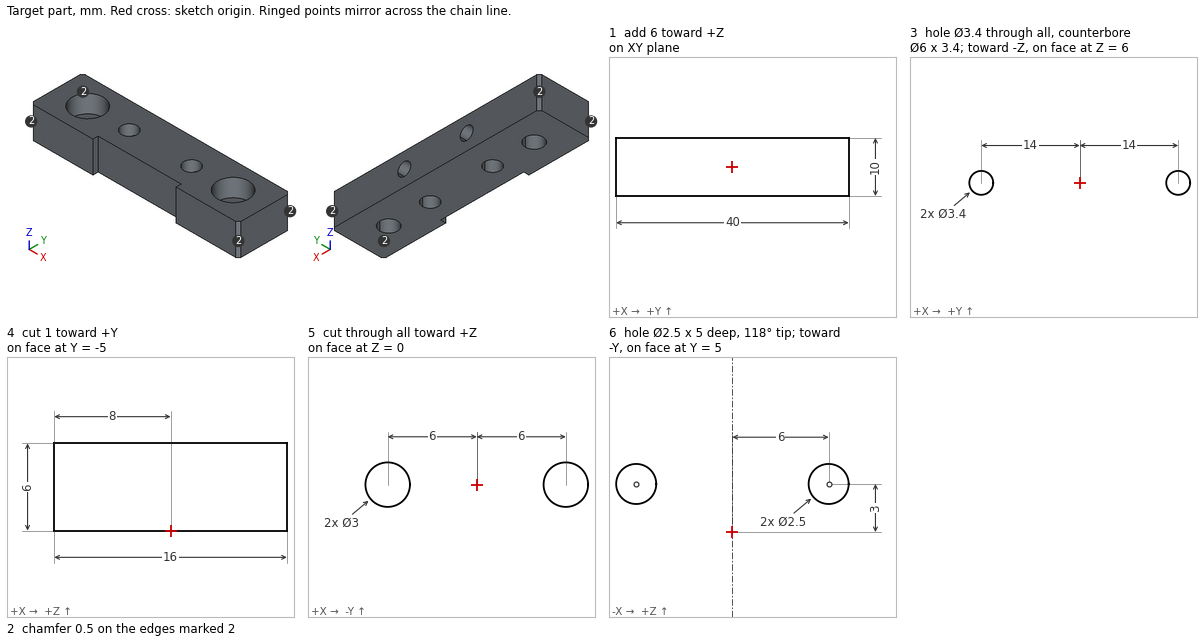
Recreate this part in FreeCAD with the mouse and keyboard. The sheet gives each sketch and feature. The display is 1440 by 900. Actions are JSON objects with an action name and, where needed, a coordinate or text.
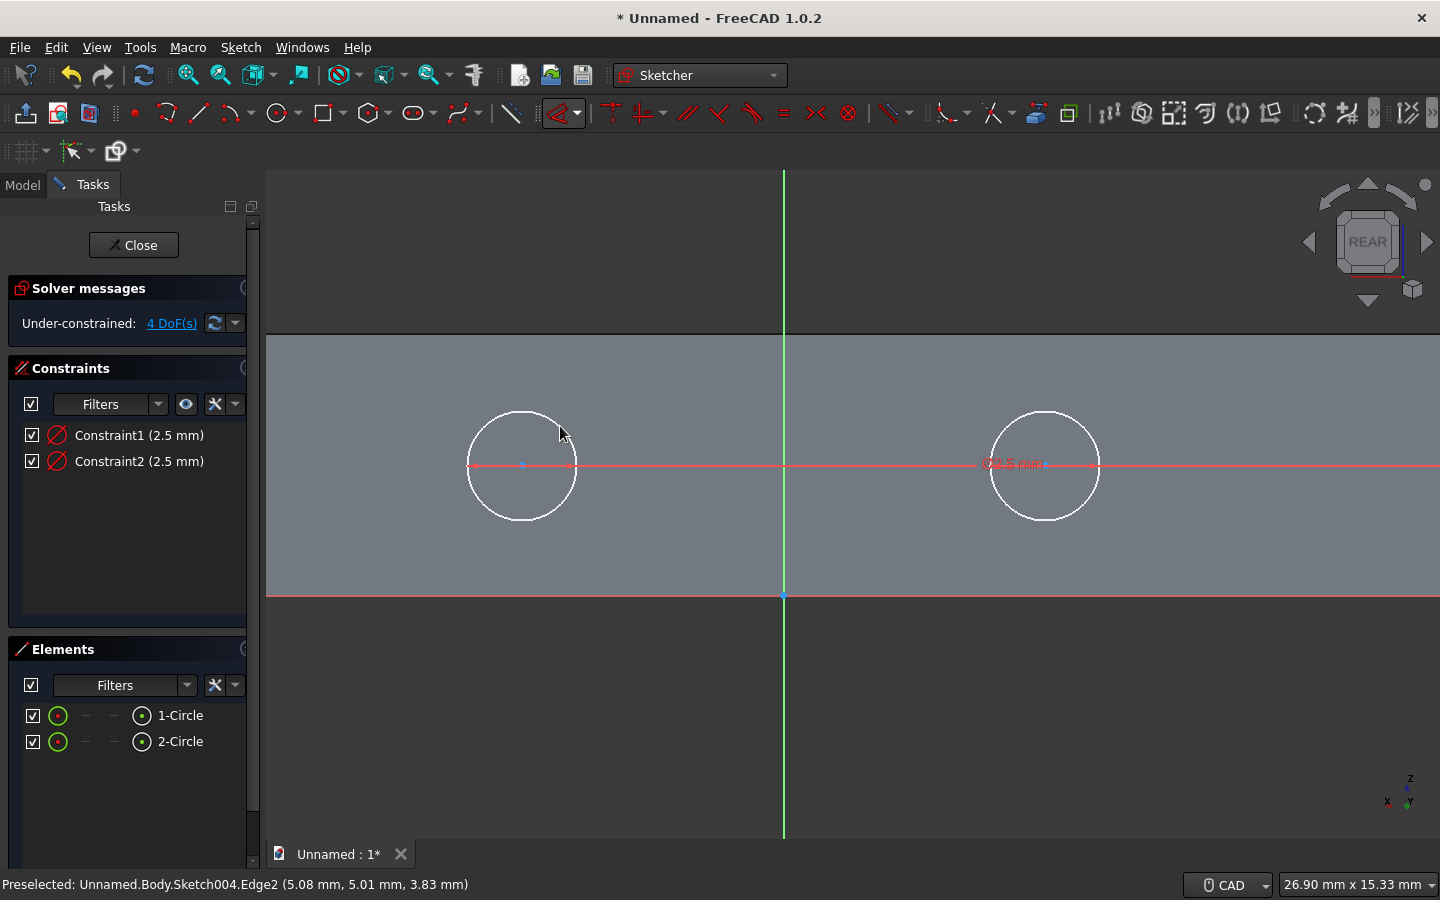
{"action": "left_click", "coordinate": [1045, 466]}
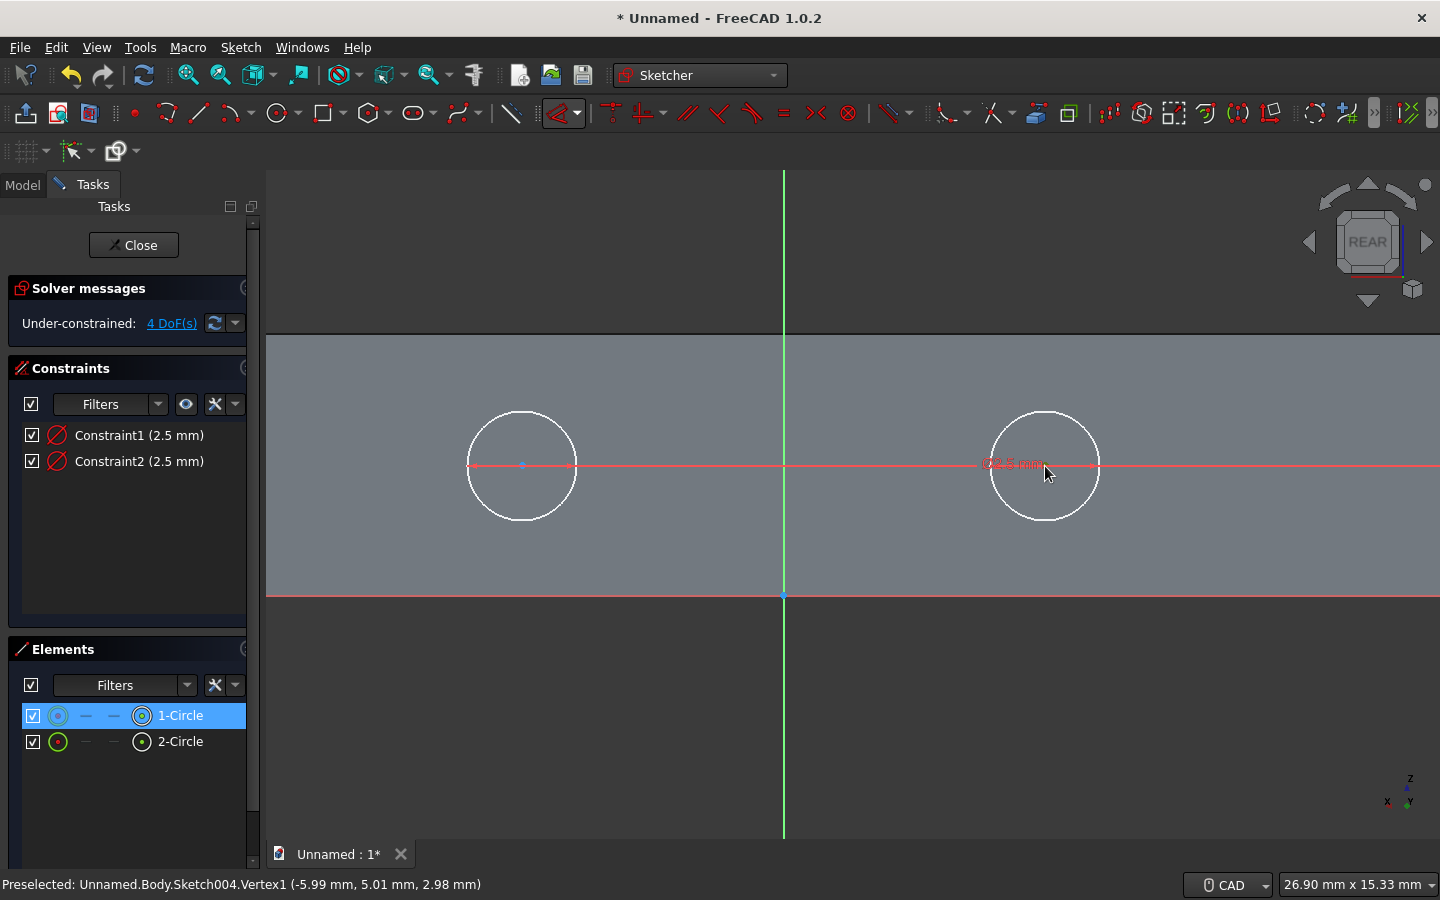
{"action": "left_click", "coordinate": [522, 466]}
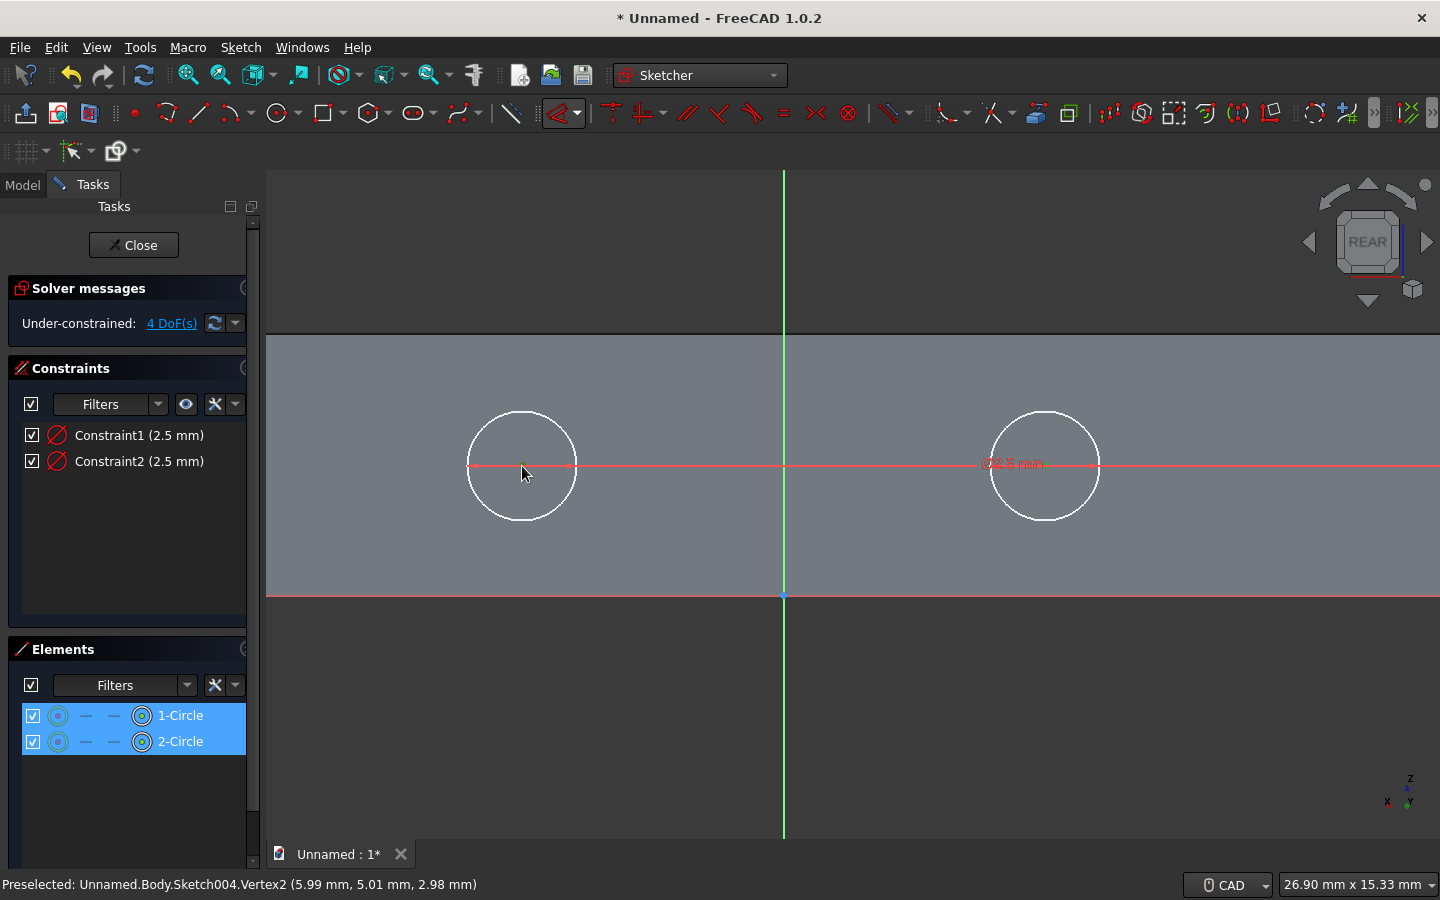
{"action": "left_click", "coordinate": [784, 767]}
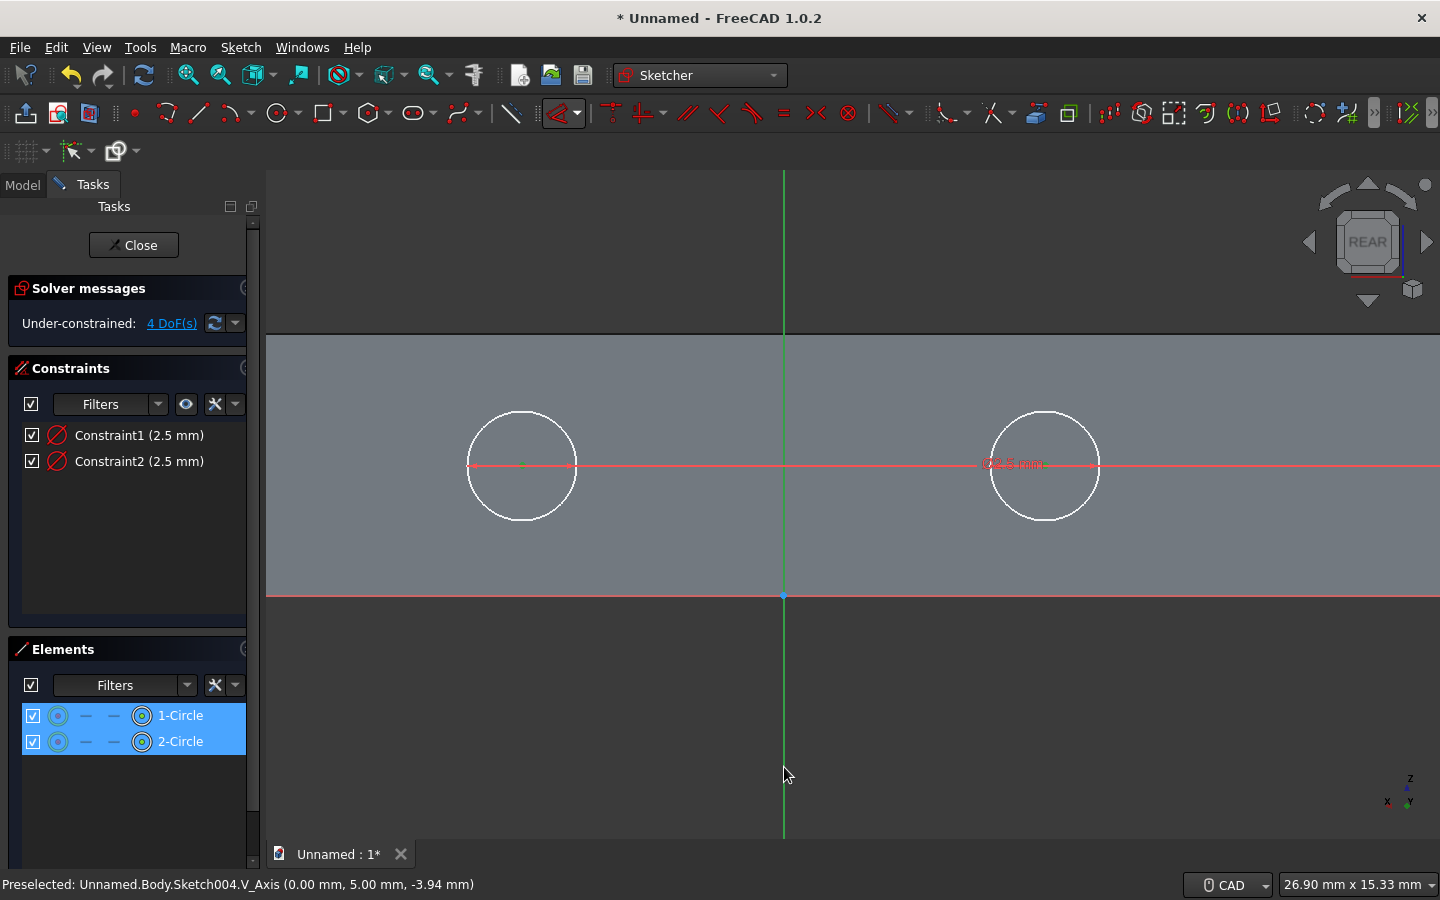
{"action": "left_click", "coordinate": [816, 114]}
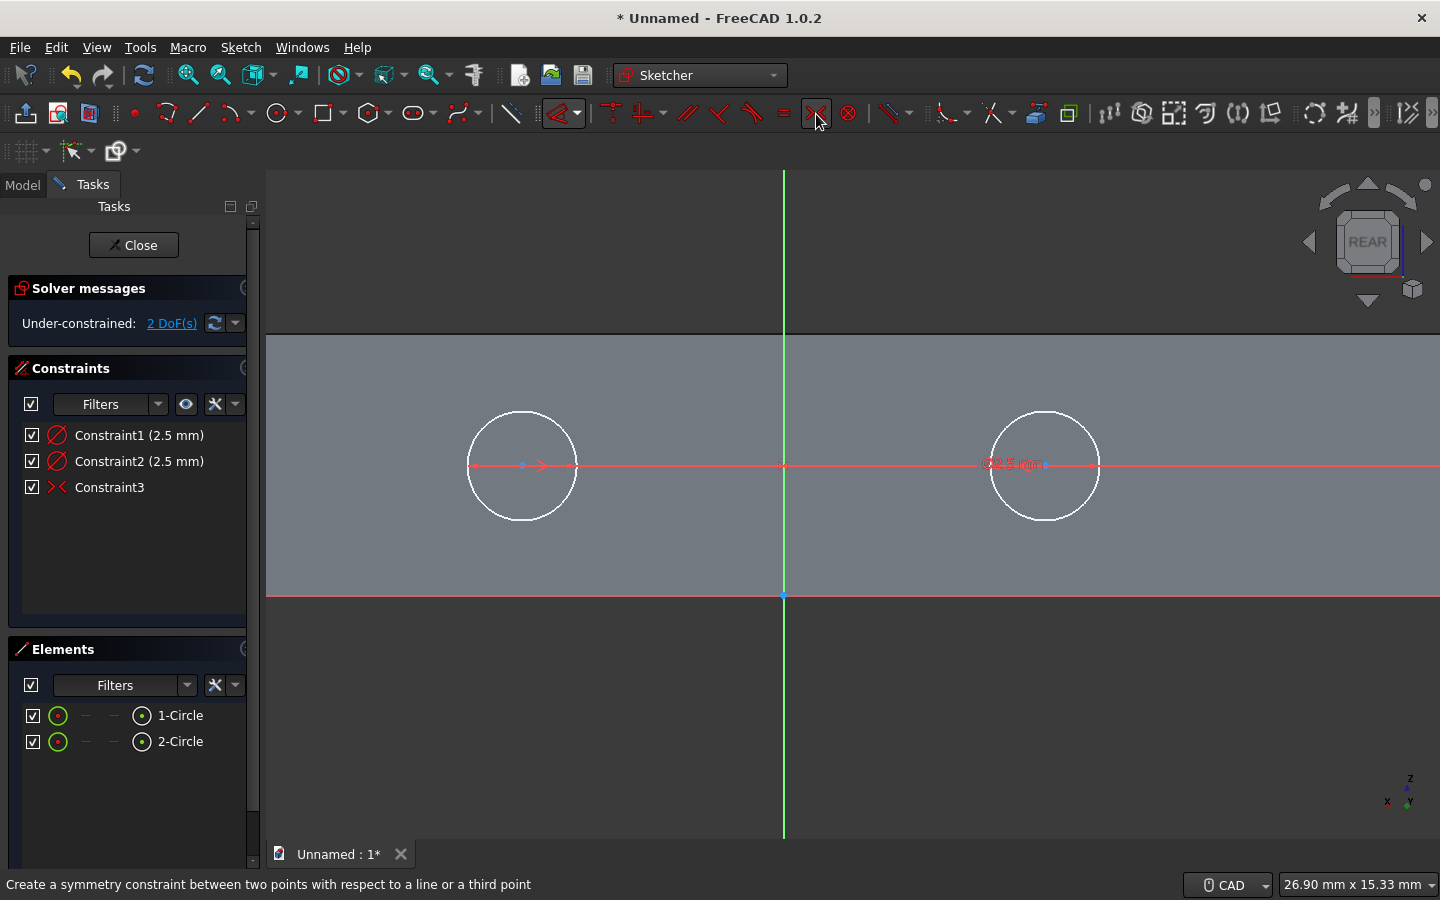
{"action": "left_click", "coordinate": [1045, 466]}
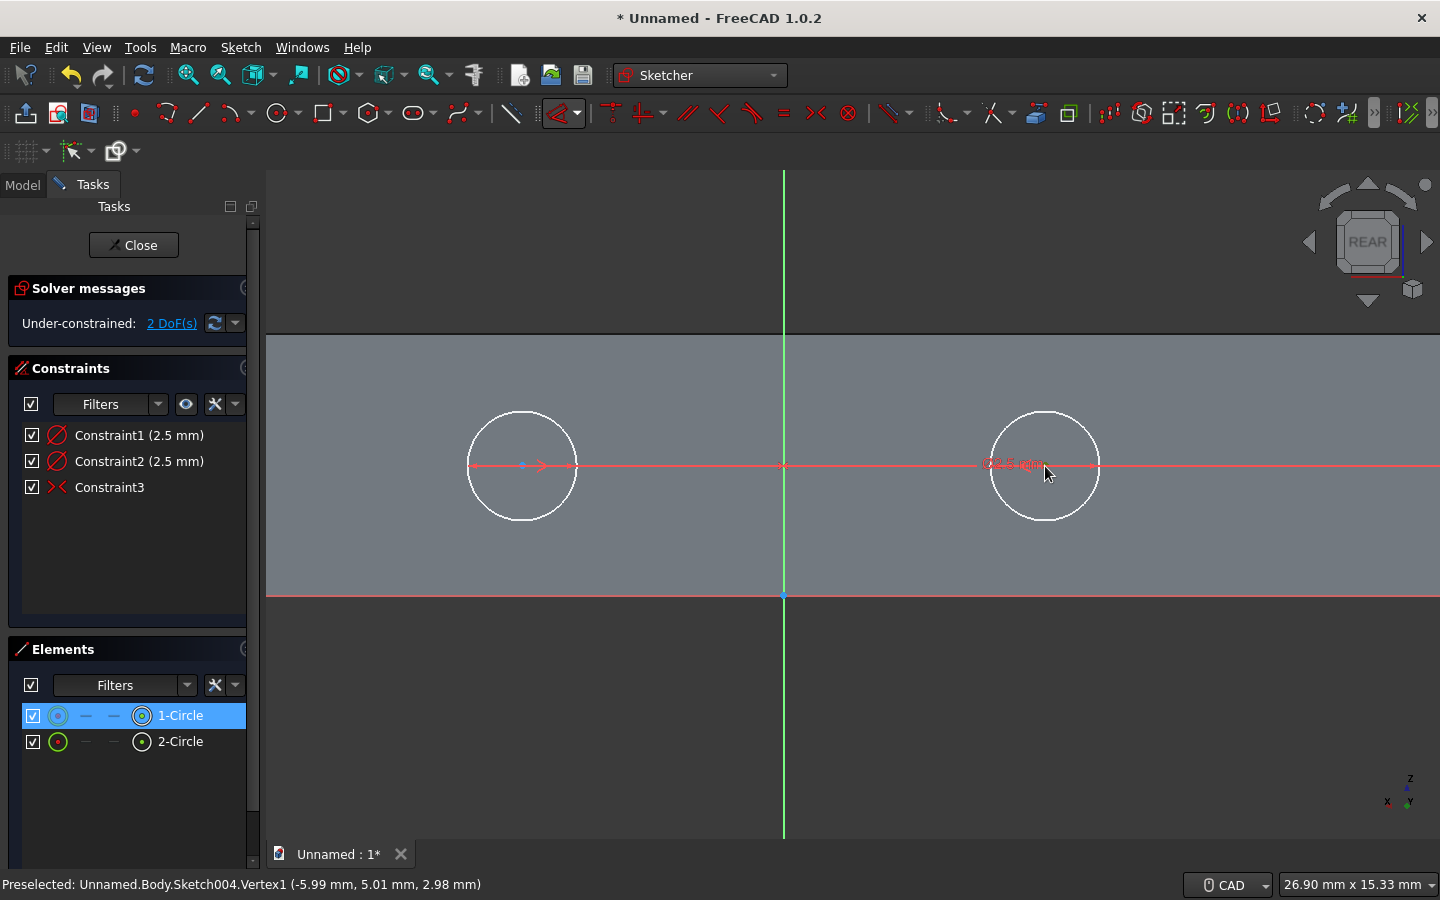
{"action": "key", "text": "l"}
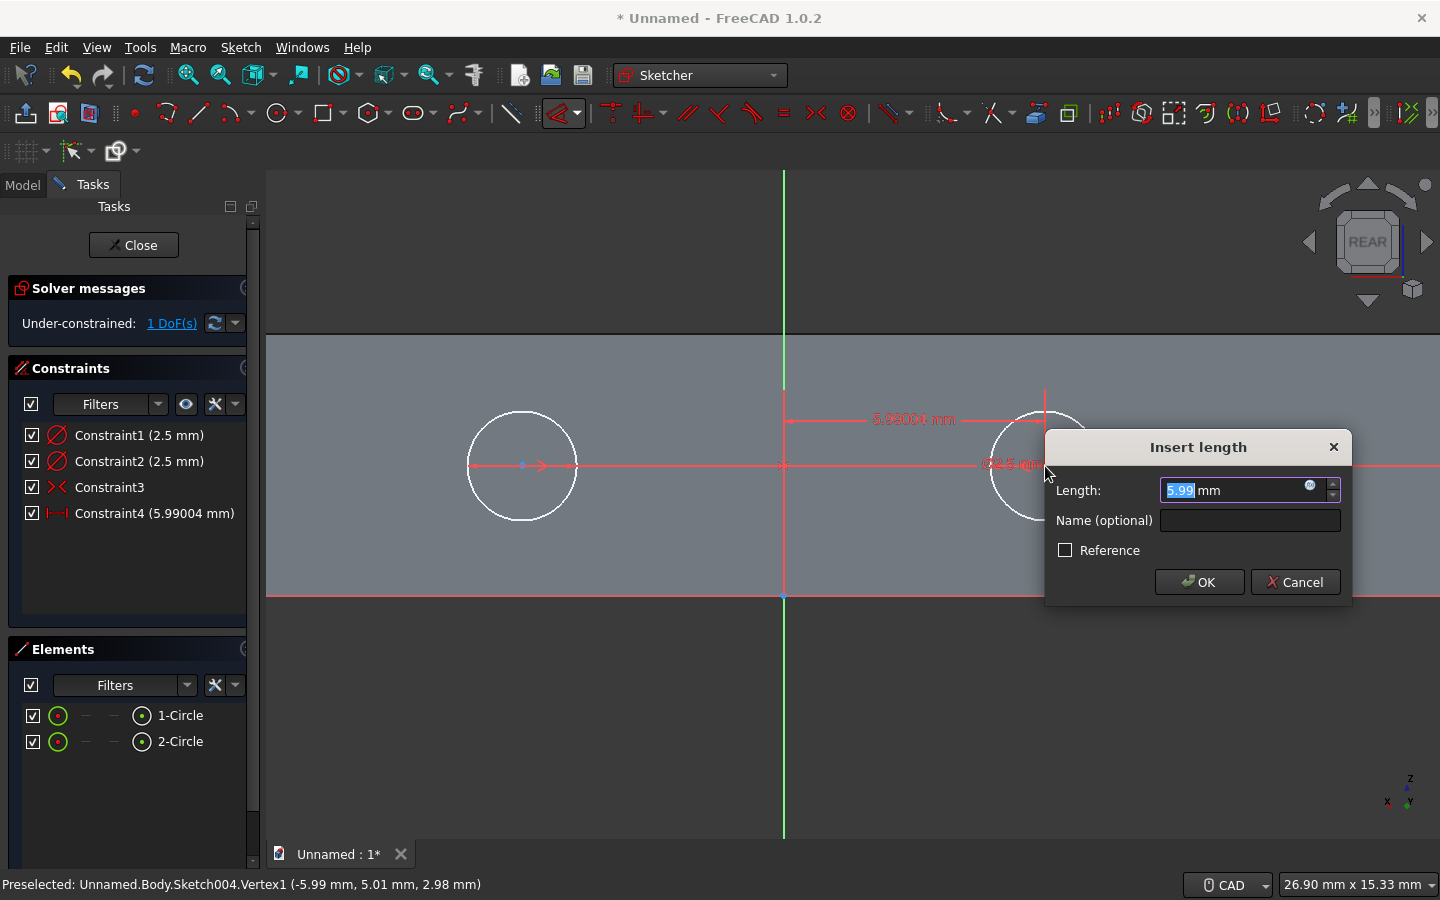
{"action": "type", "text": "6"}
{"action": "key", "text": "Return"}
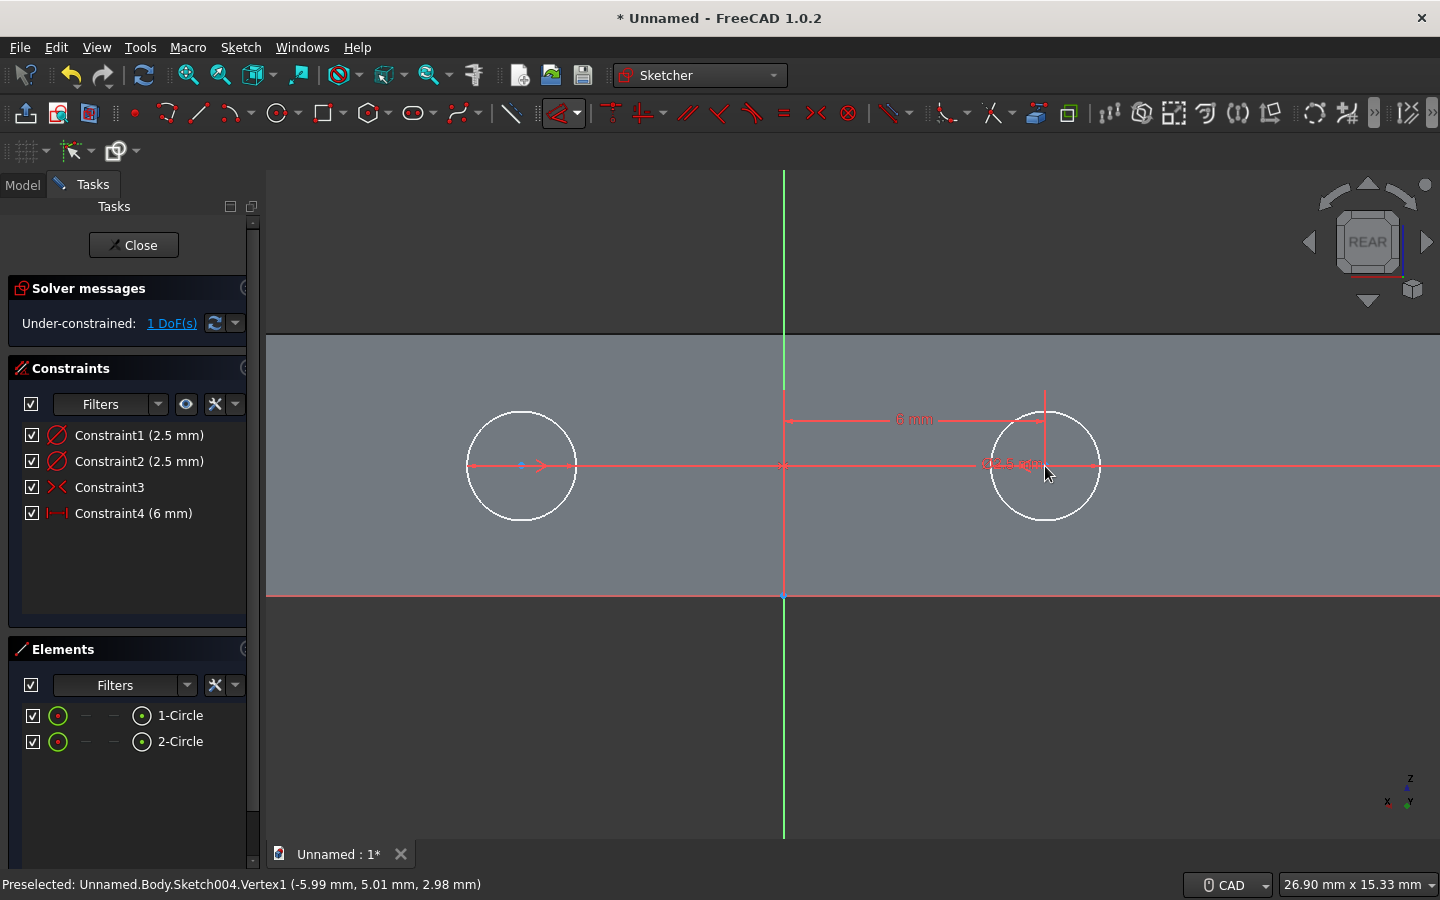
{"action": "left_click", "coordinate": [1045, 466]}